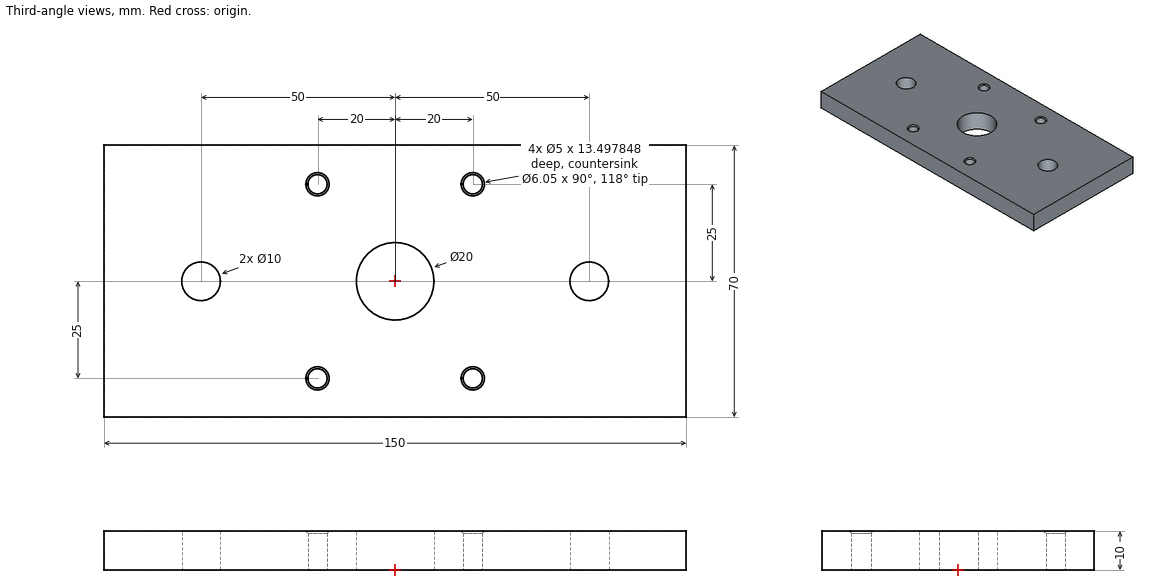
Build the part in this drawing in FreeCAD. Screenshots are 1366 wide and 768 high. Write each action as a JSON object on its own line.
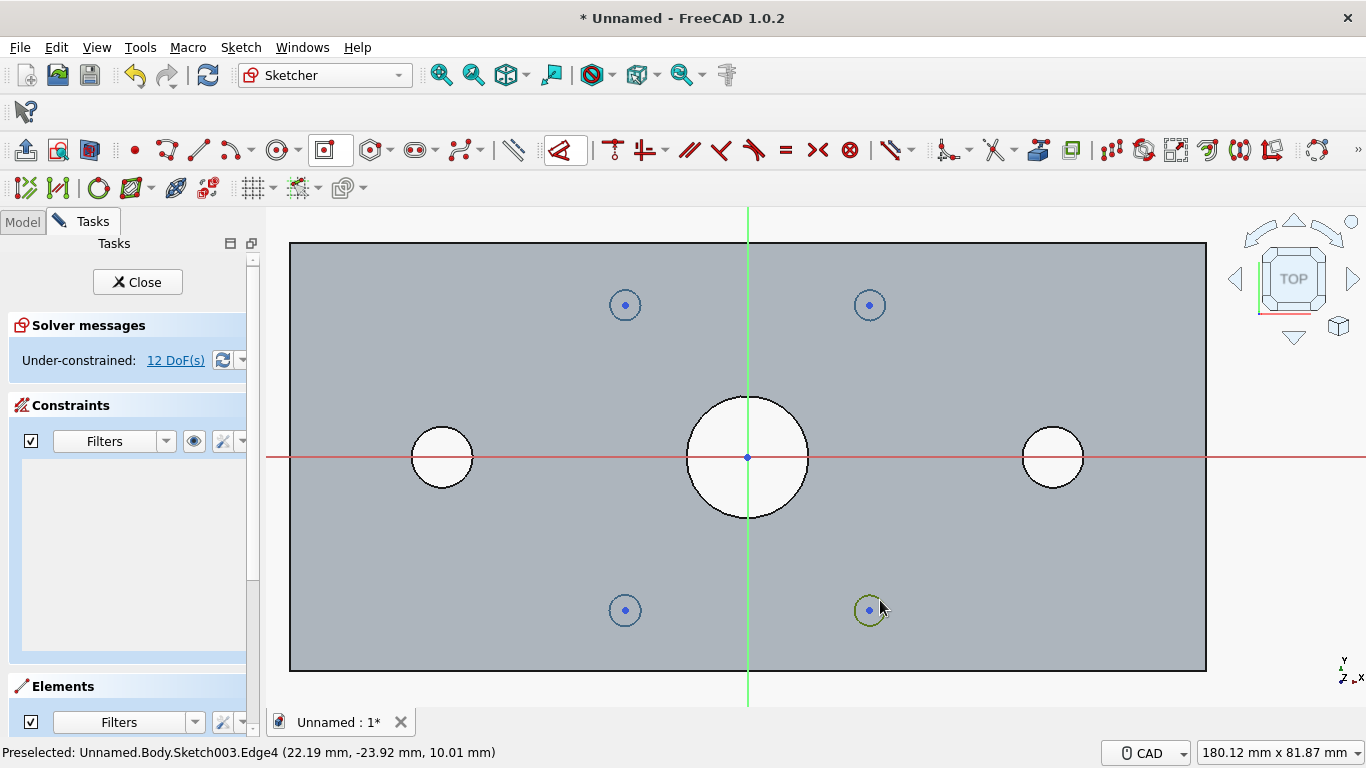
{"action": "left_click", "coordinate": [786, 150]}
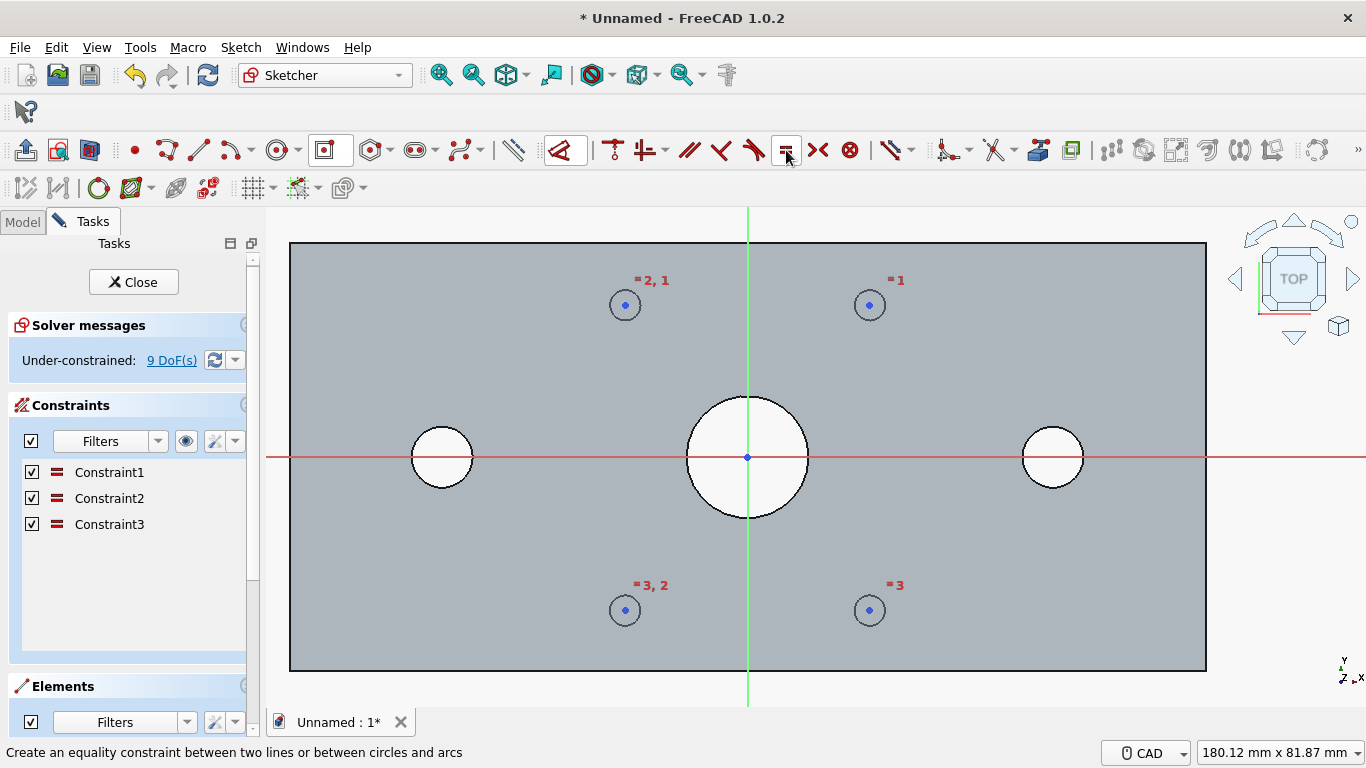
{"action": "left_click", "coordinate": [870, 305]}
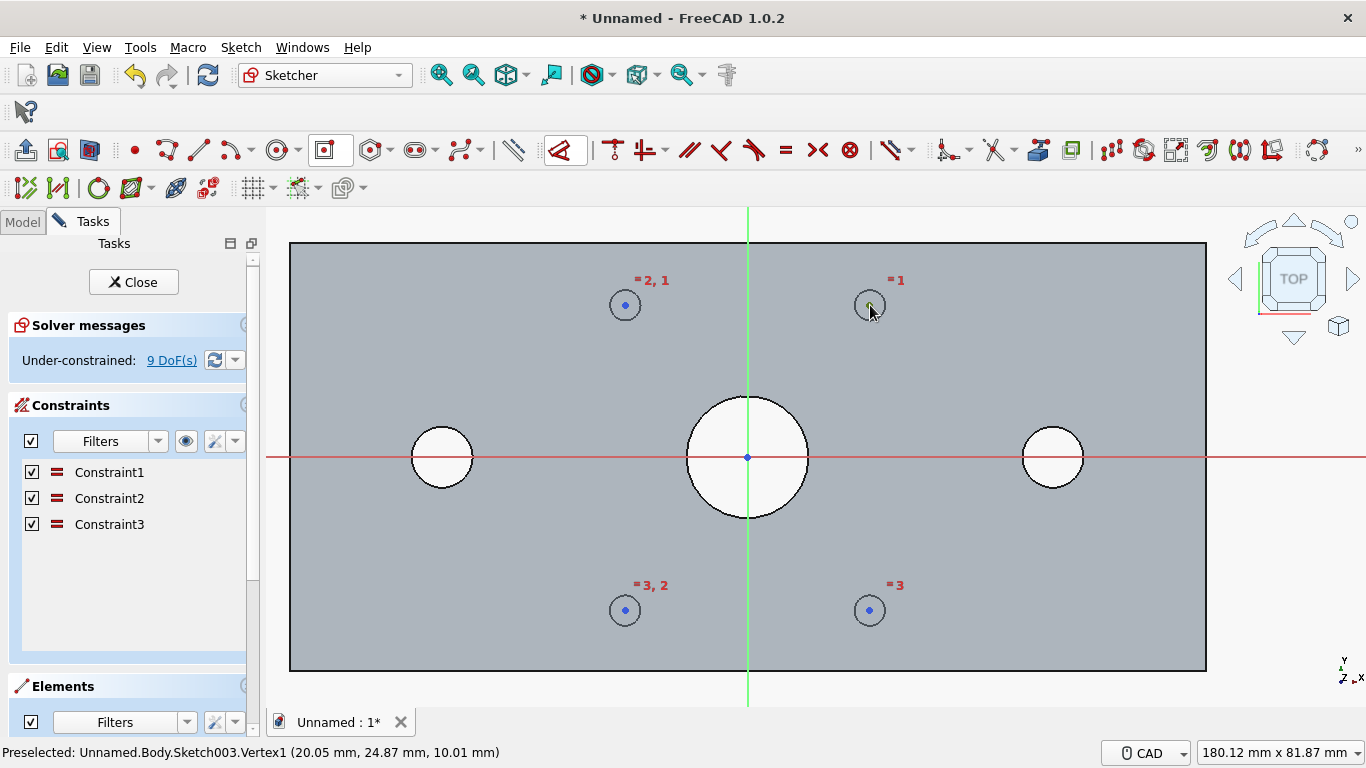
{"action": "left_click", "coordinate": [625, 305]}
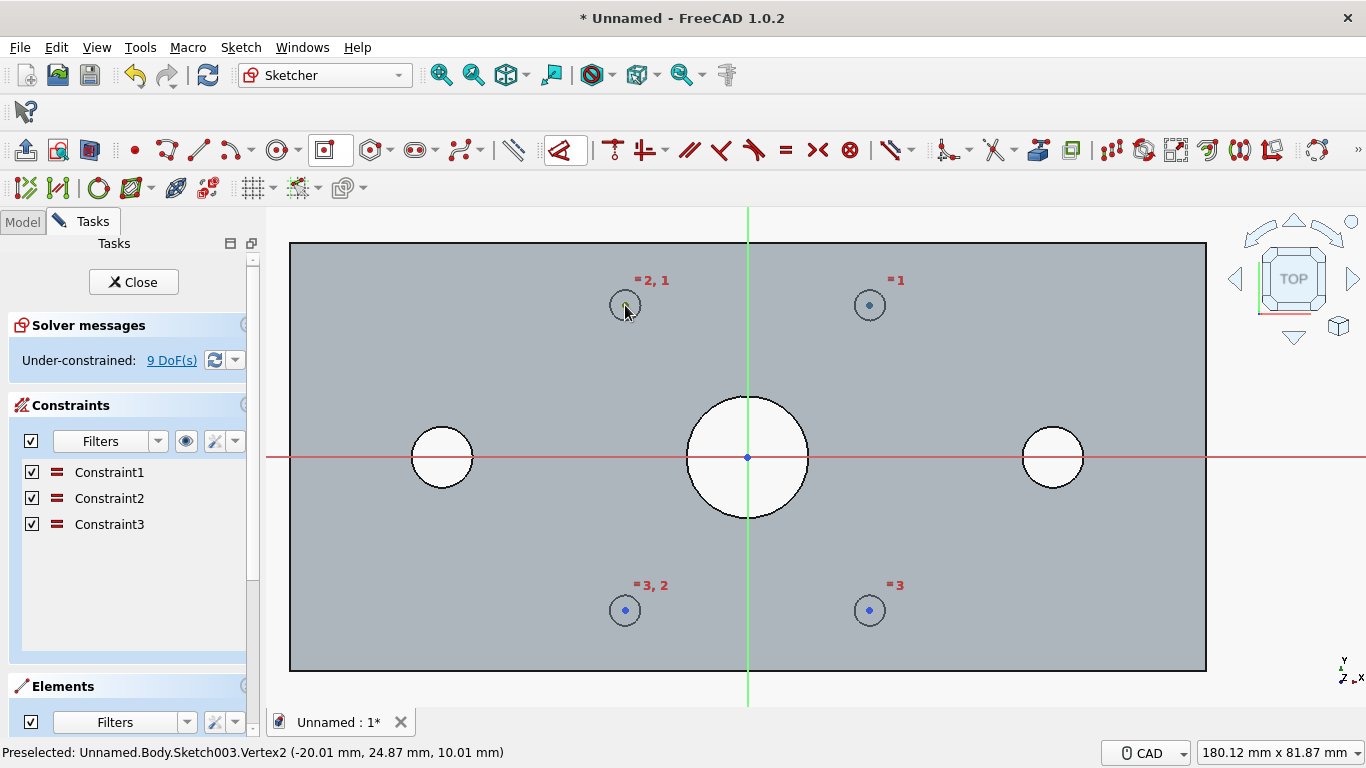
{"action": "left_click", "coordinate": [668, 150]}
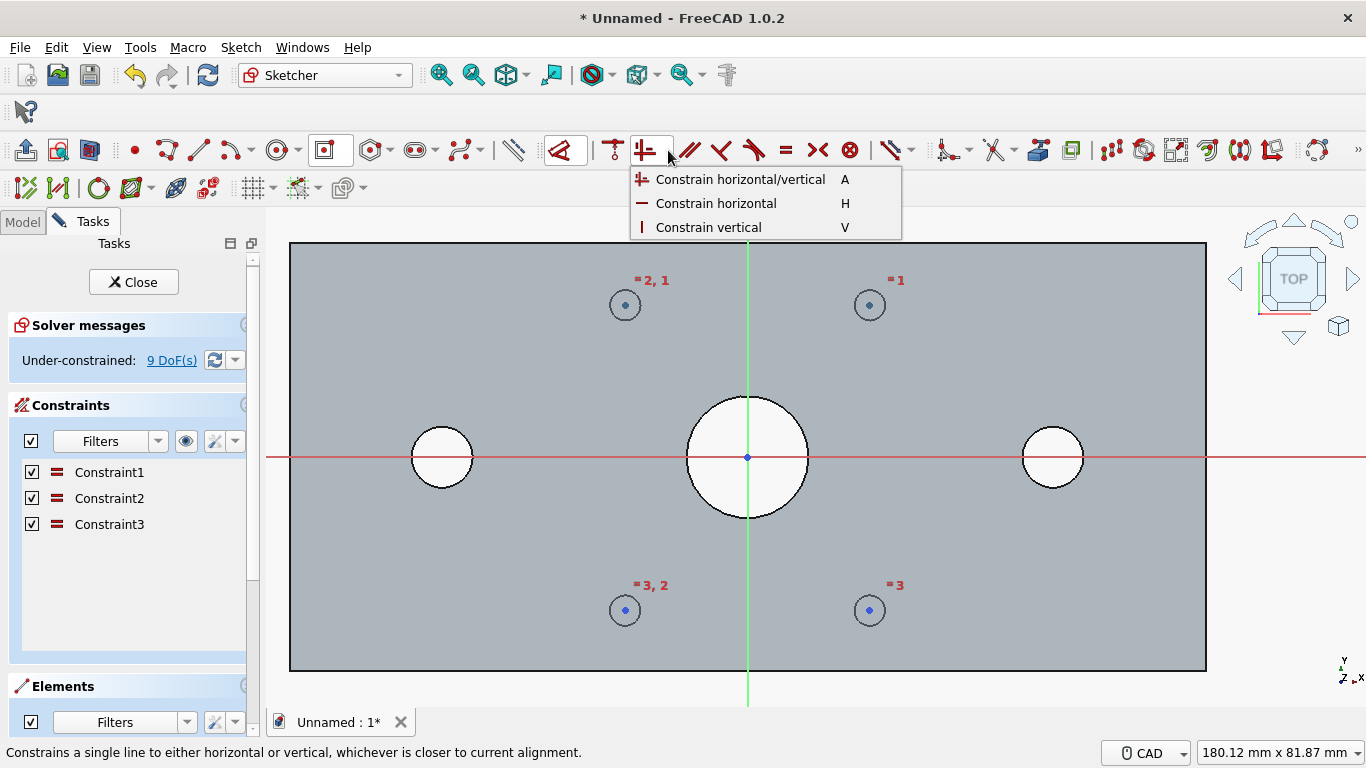
{"action": "left_click", "coordinate": [766, 203]}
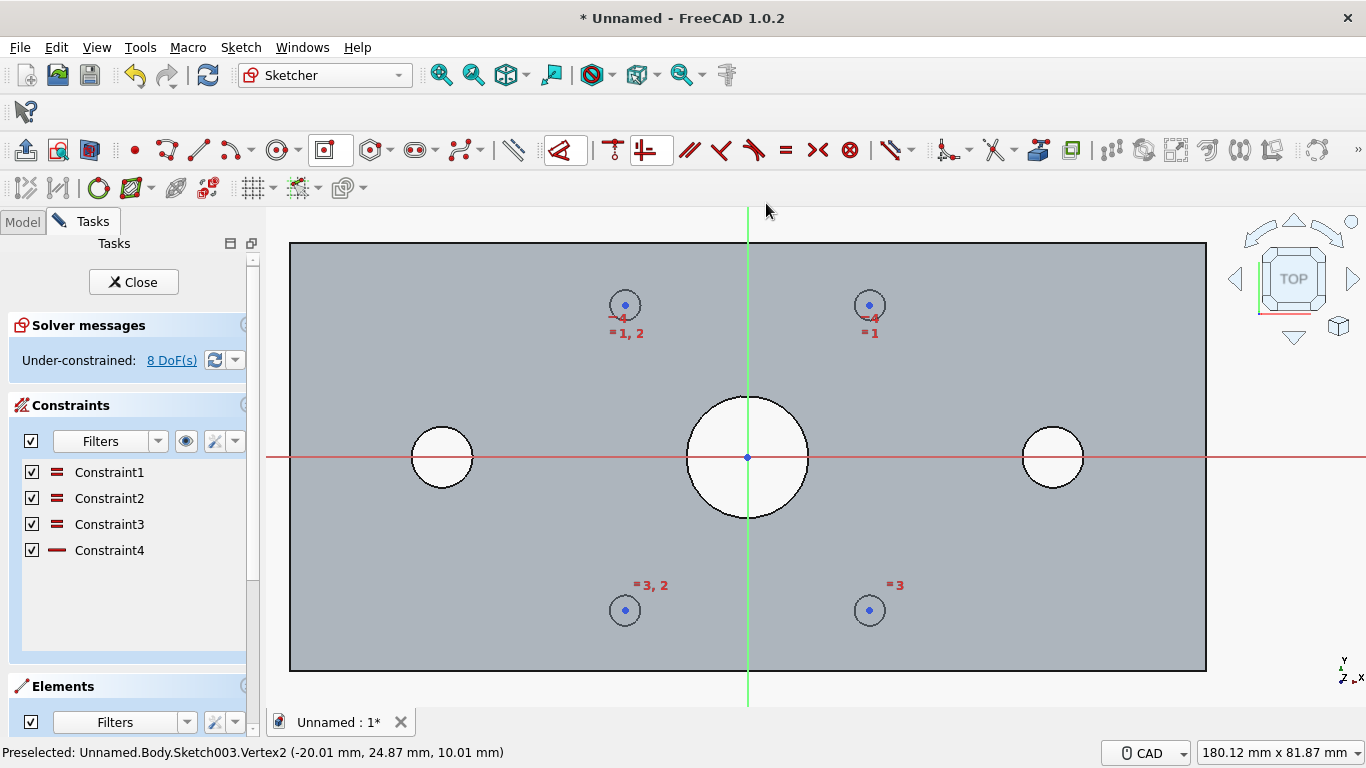
{"action": "left_click", "coordinate": [625, 305]}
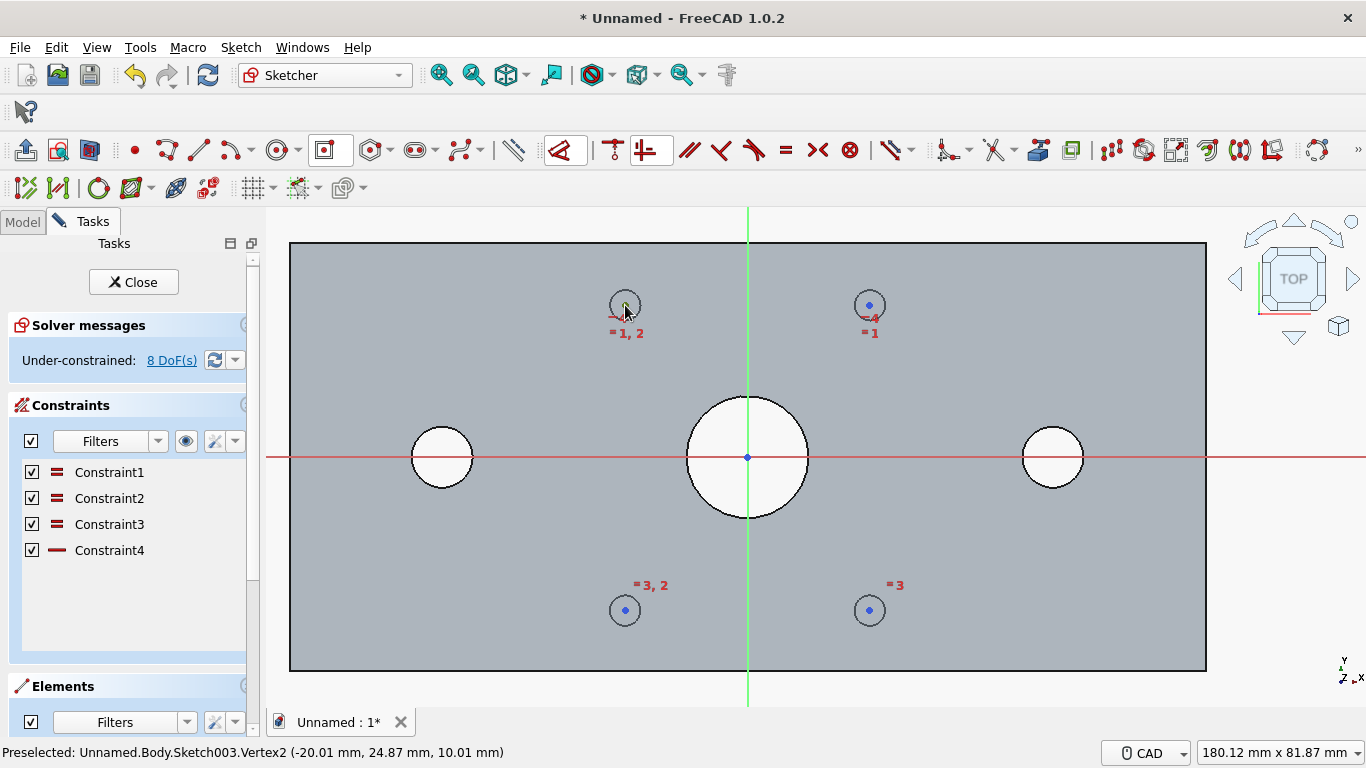
{"action": "left_click", "coordinate": [625, 611]}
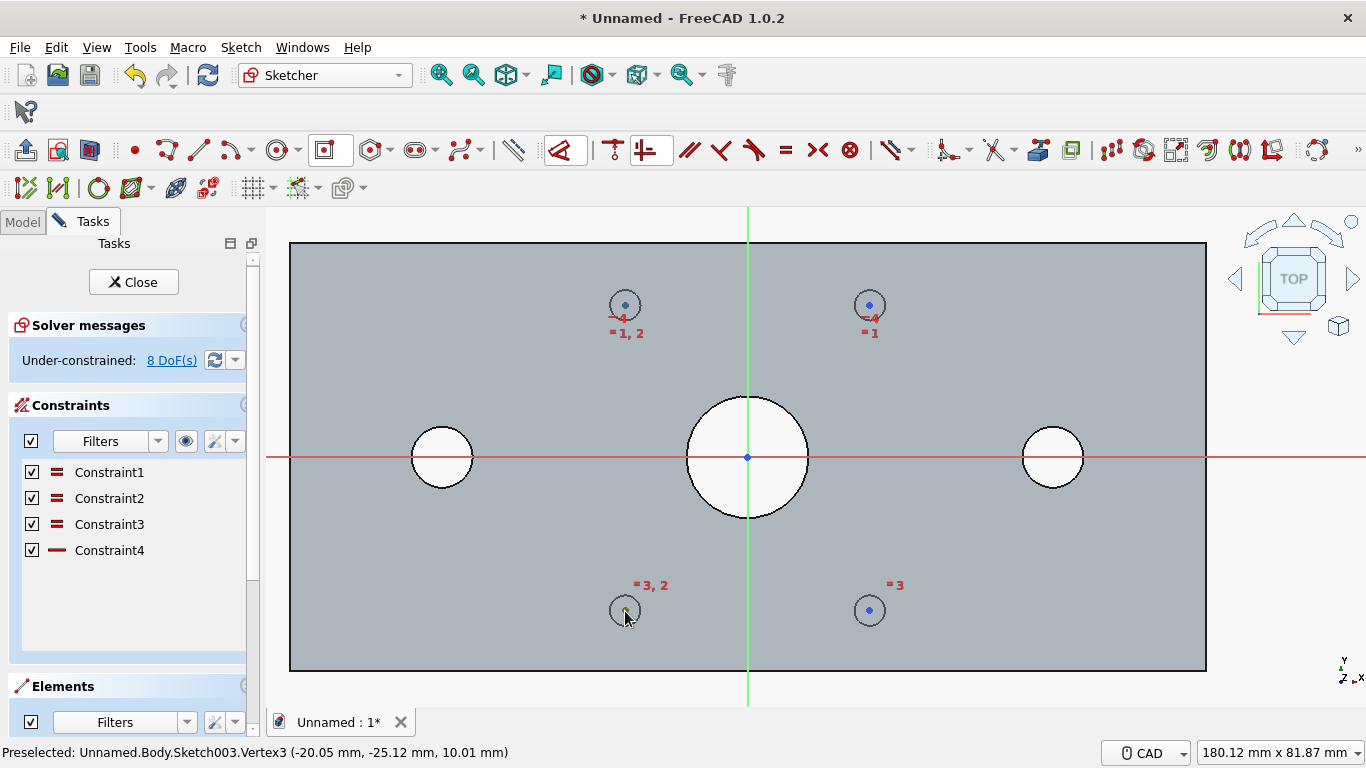
{"action": "left_click", "coordinate": [668, 150]}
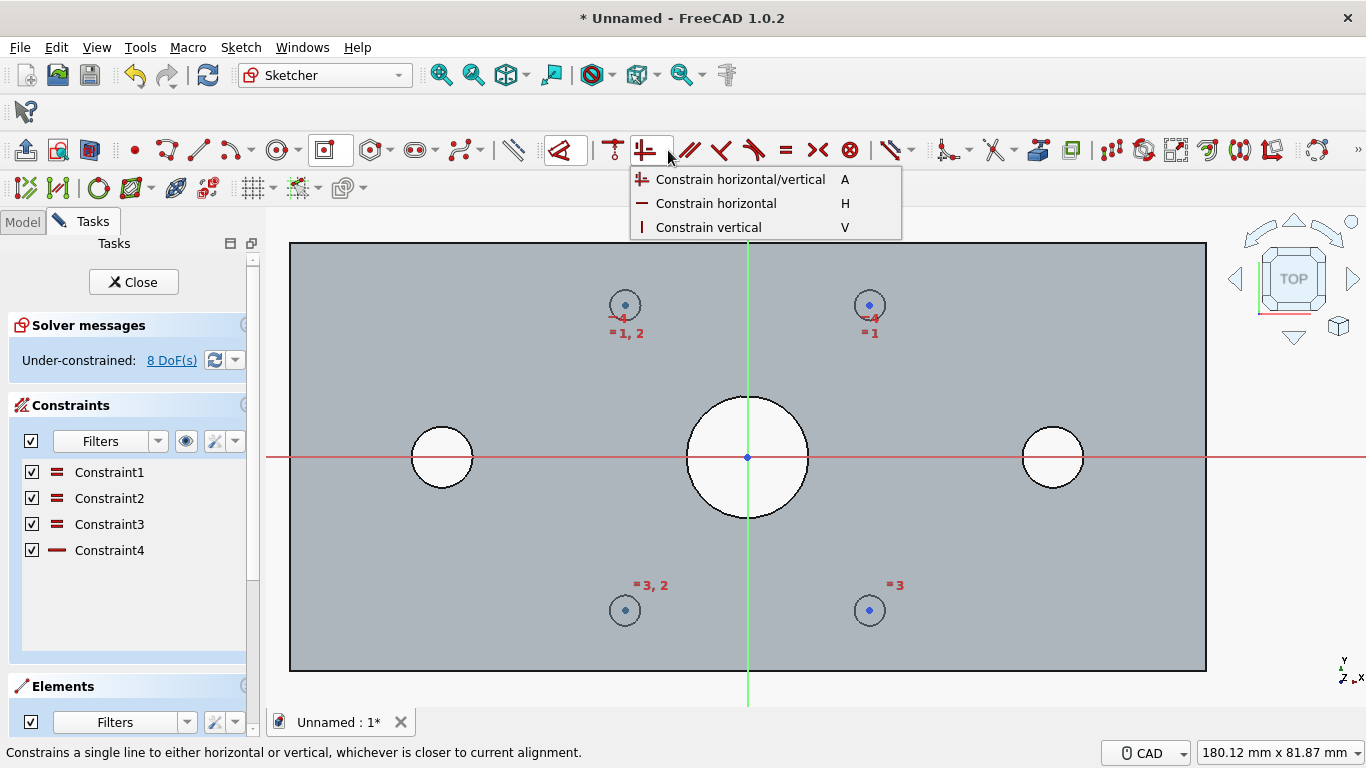
{"action": "left_click", "coordinate": [766, 227]}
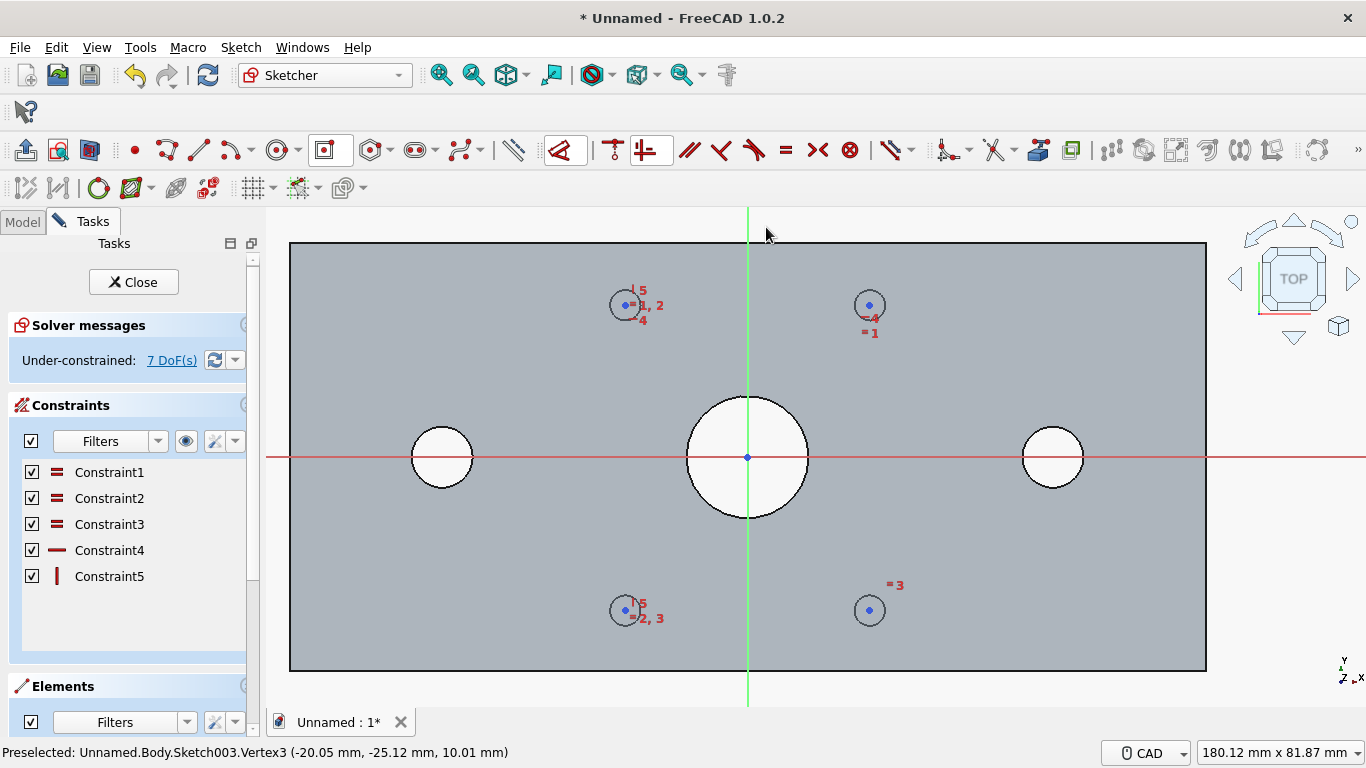
{"action": "left_click", "coordinate": [870, 305]}